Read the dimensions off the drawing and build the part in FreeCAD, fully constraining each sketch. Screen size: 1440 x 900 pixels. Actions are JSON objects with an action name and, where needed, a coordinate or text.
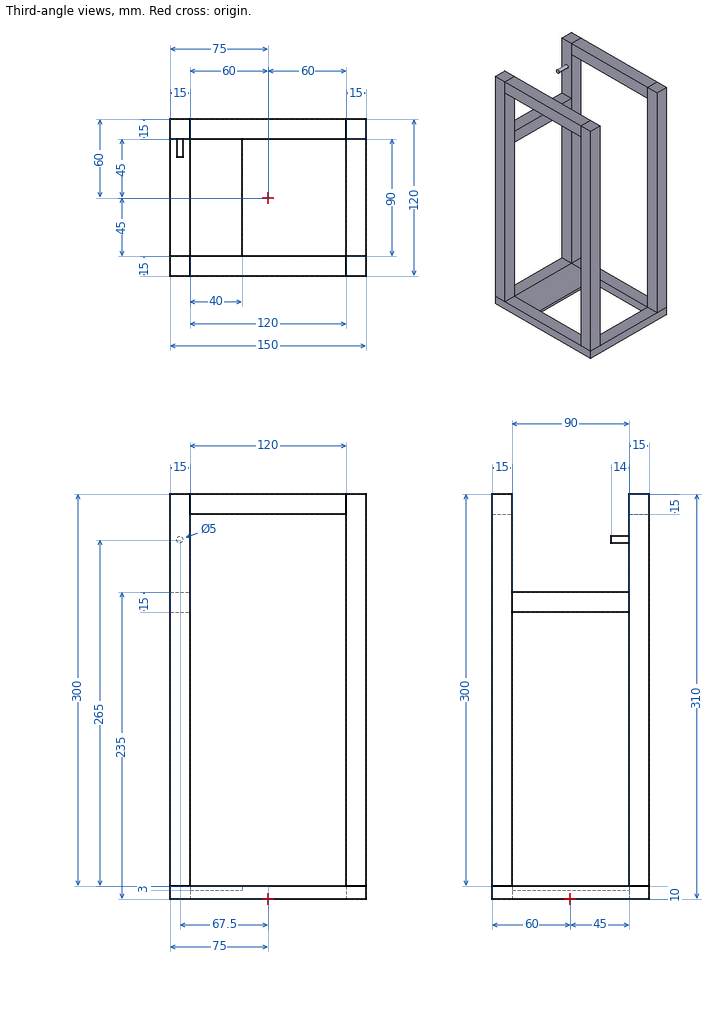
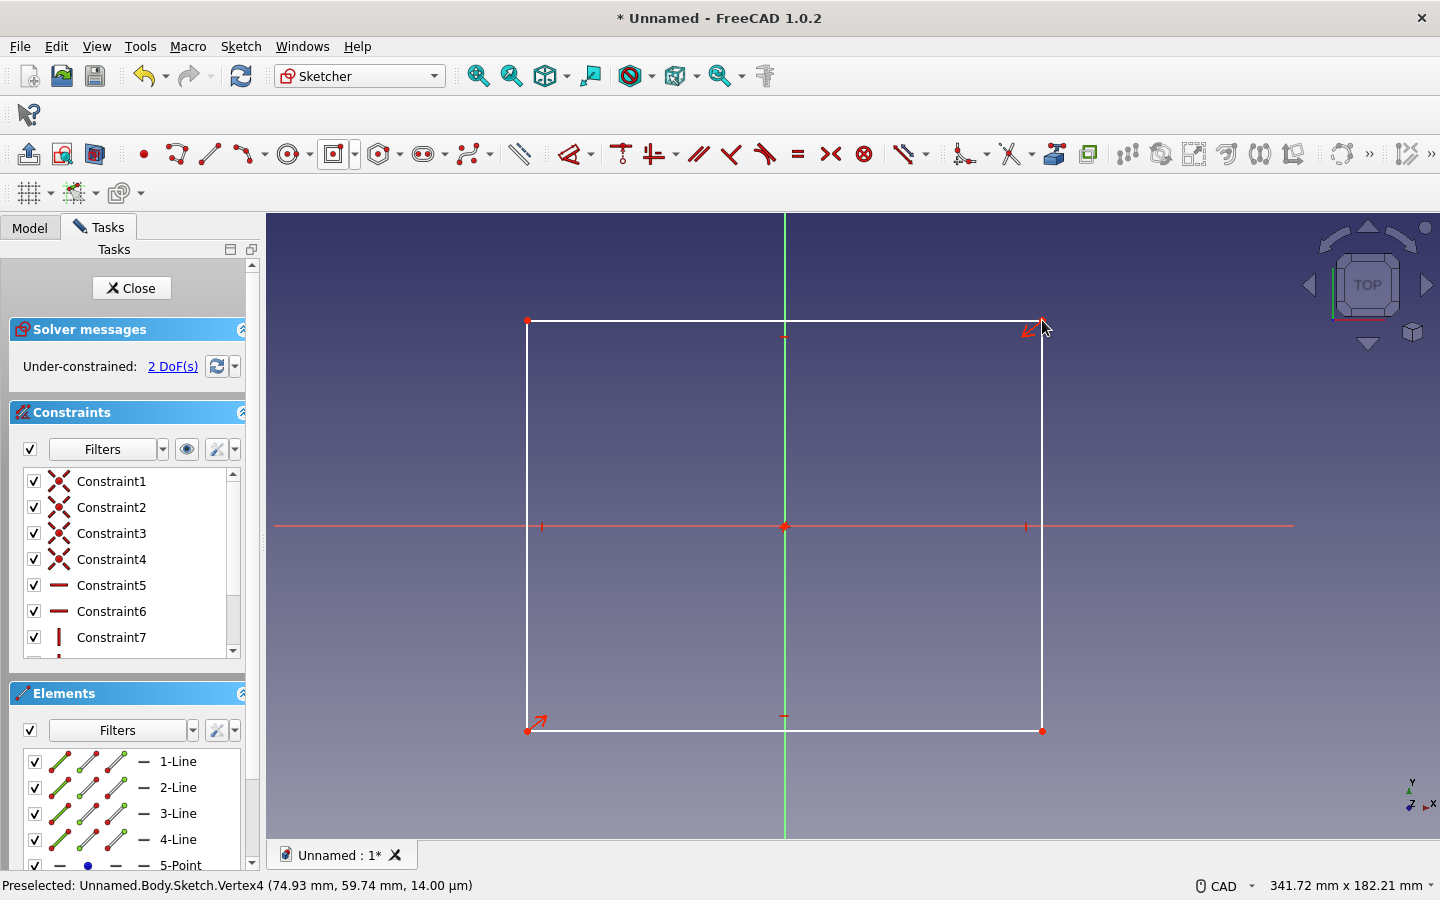
{"action": "left_click", "coordinate": [568, 154]}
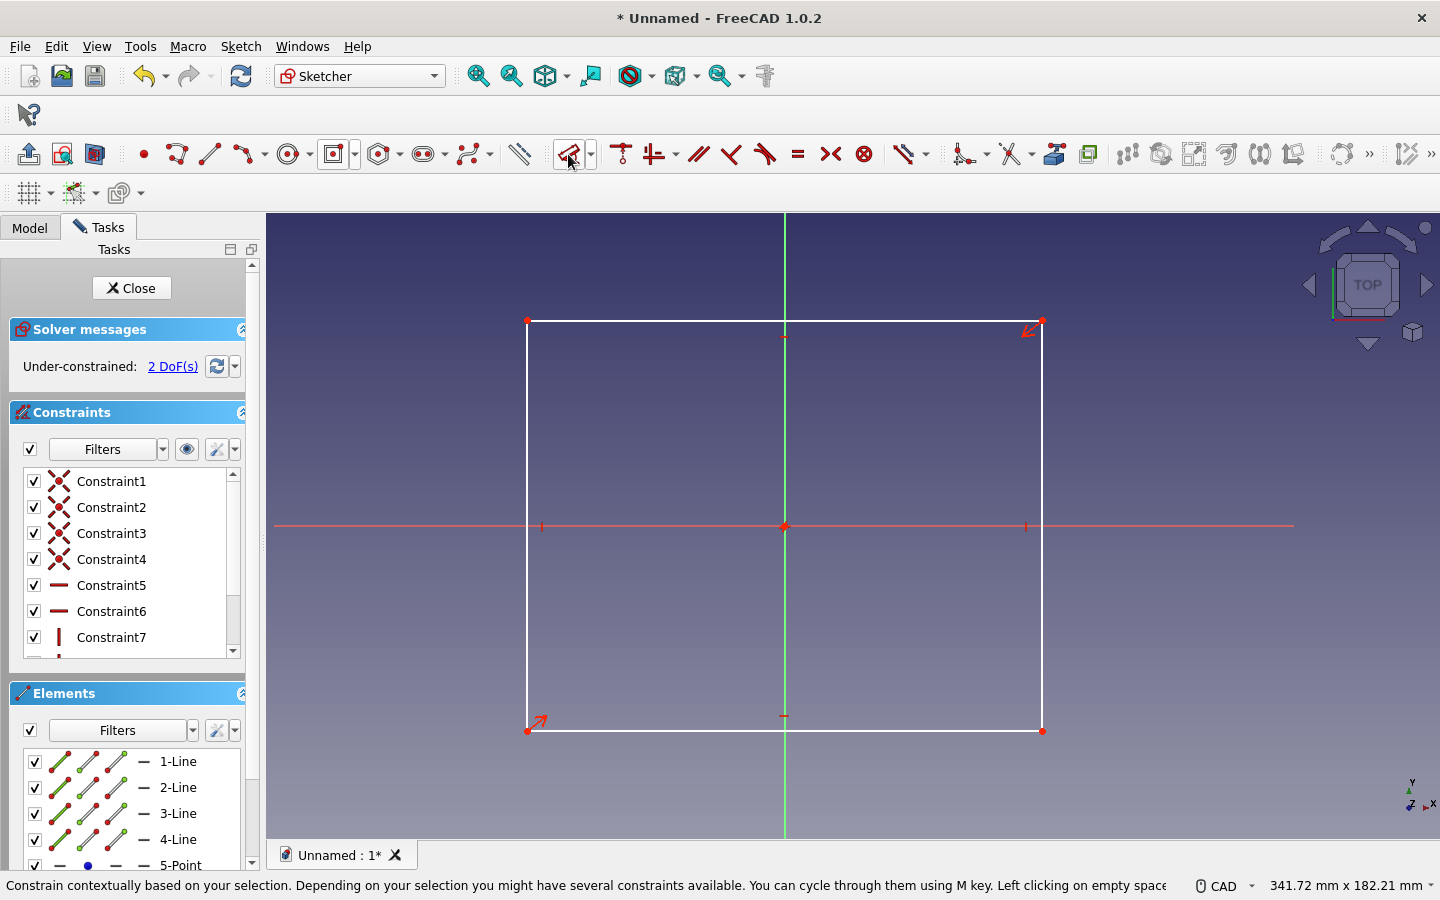
{"action": "left_click", "coordinate": [682, 731]}
{"action": "left_click", "coordinate": [666, 765]}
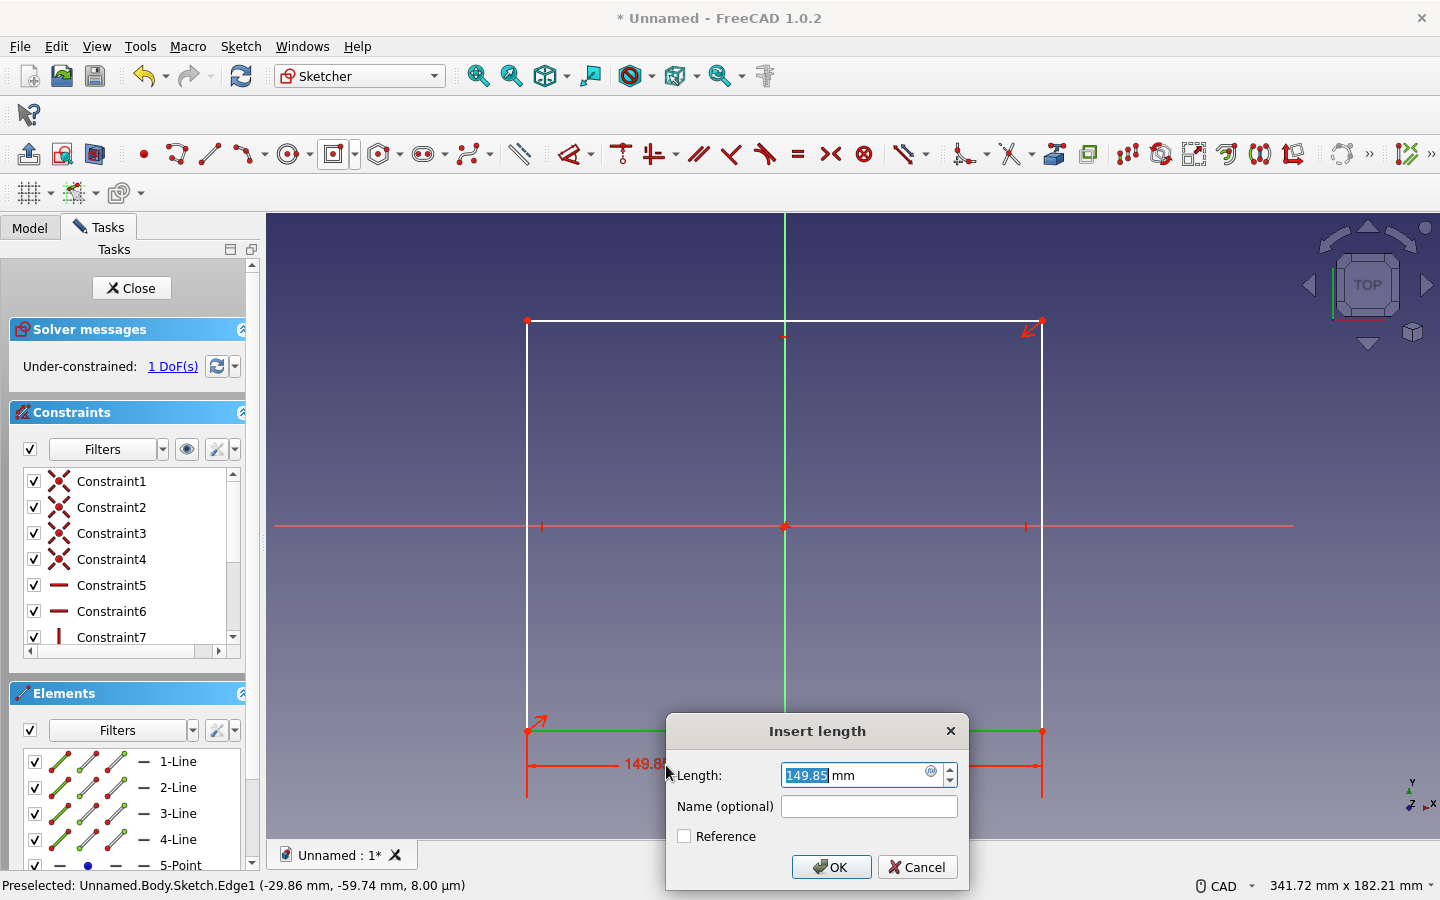
{"action": "type", "text": "150"}
{"action": "key", "text": "Return"}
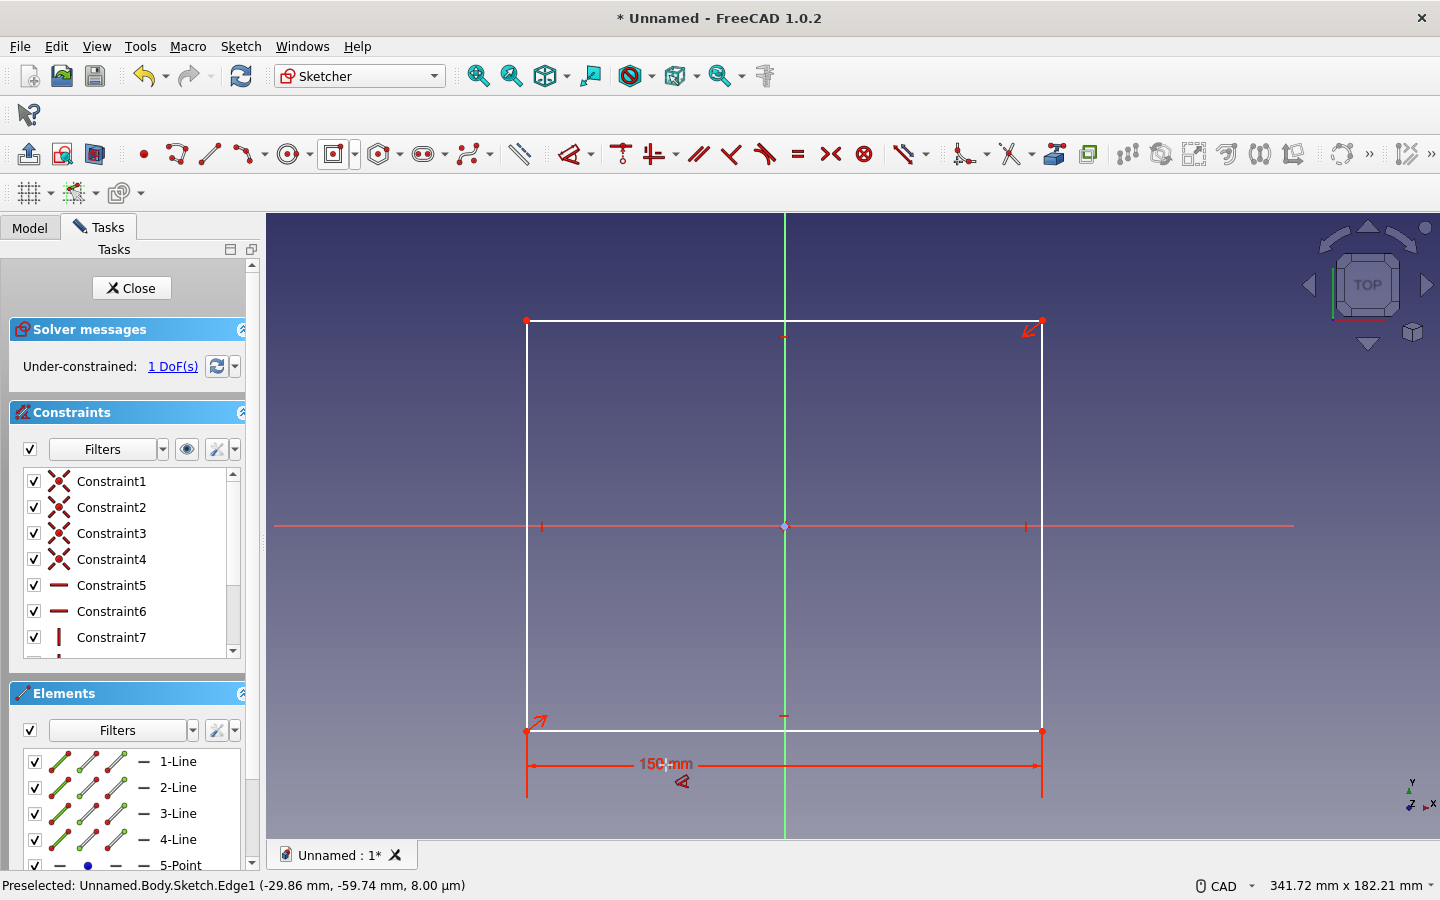
{"action": "left_click", "coordinate": [1042, 608]}
{"action": "left_click", "coordinate": [1076, 432]}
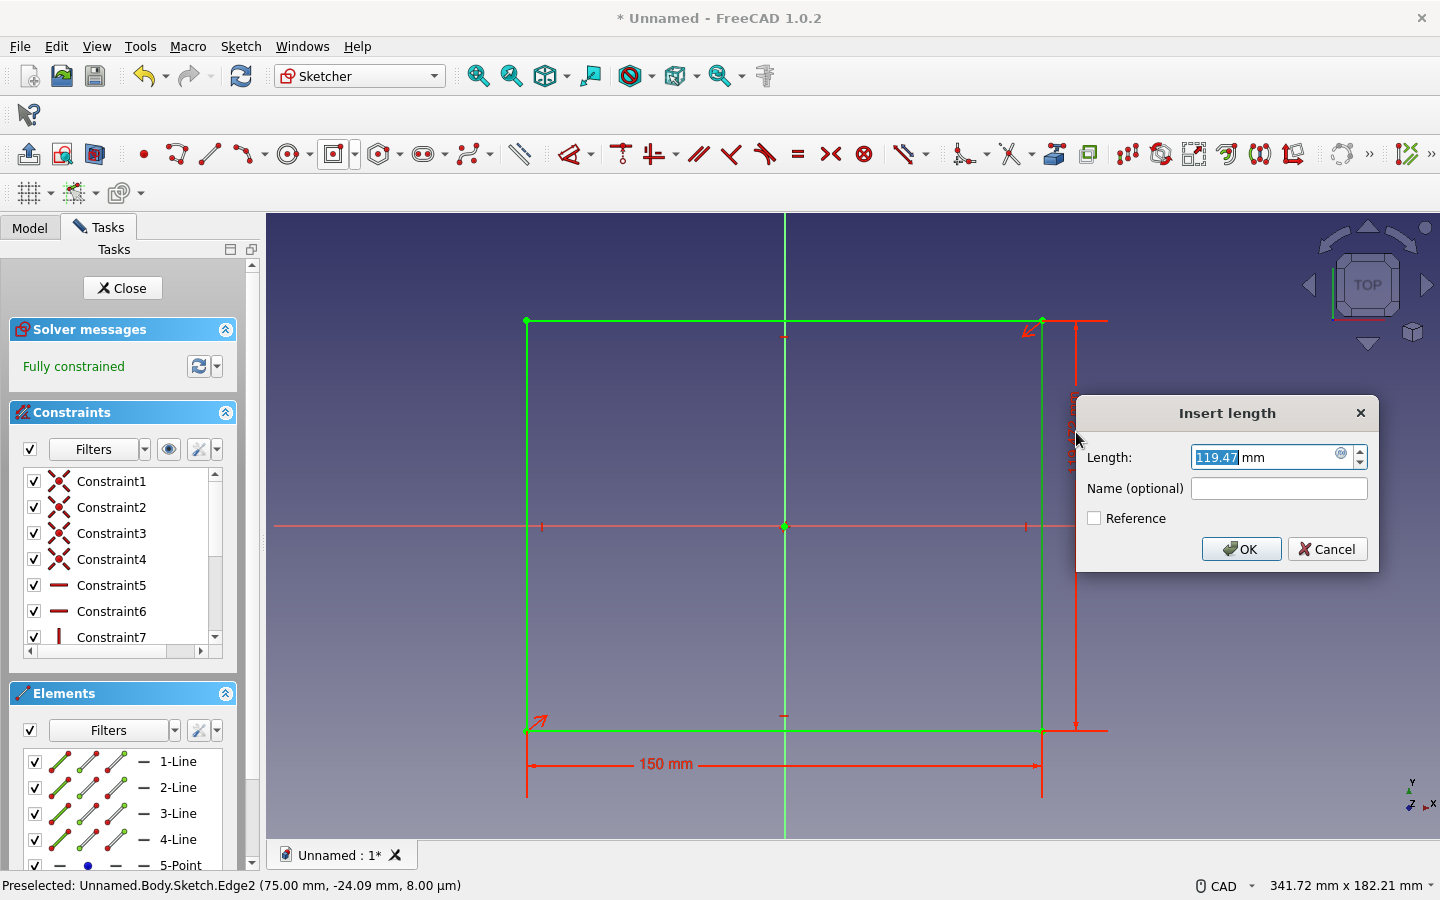
{"action": "type", "text": "120"}
{"action": "key", "text": "Return"}
{"action": "key", "text": "Escape"}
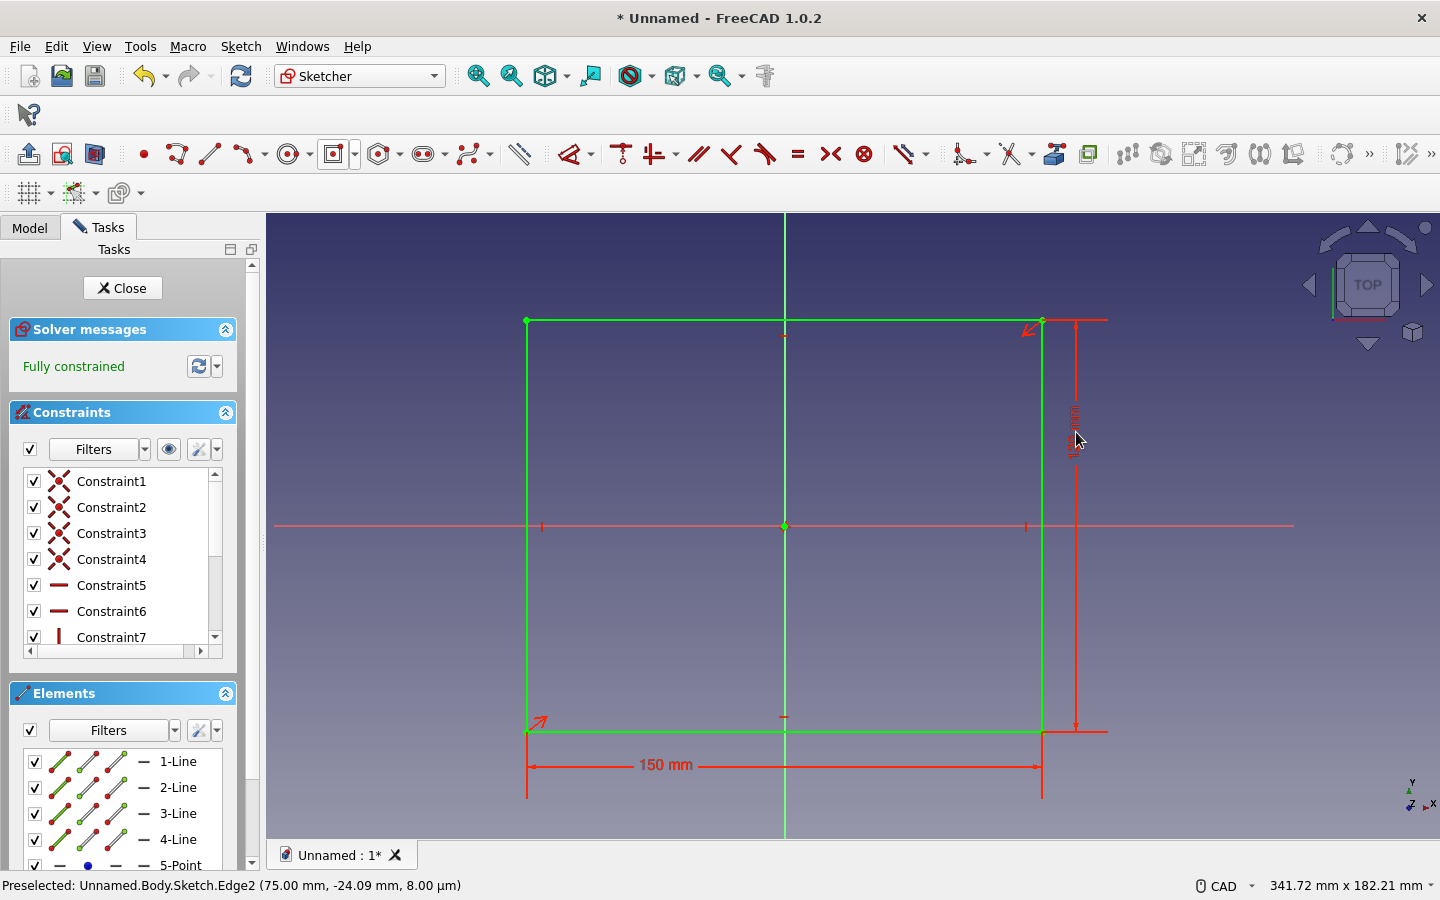
{"action": "left_click", "coordinate": [123, 288]}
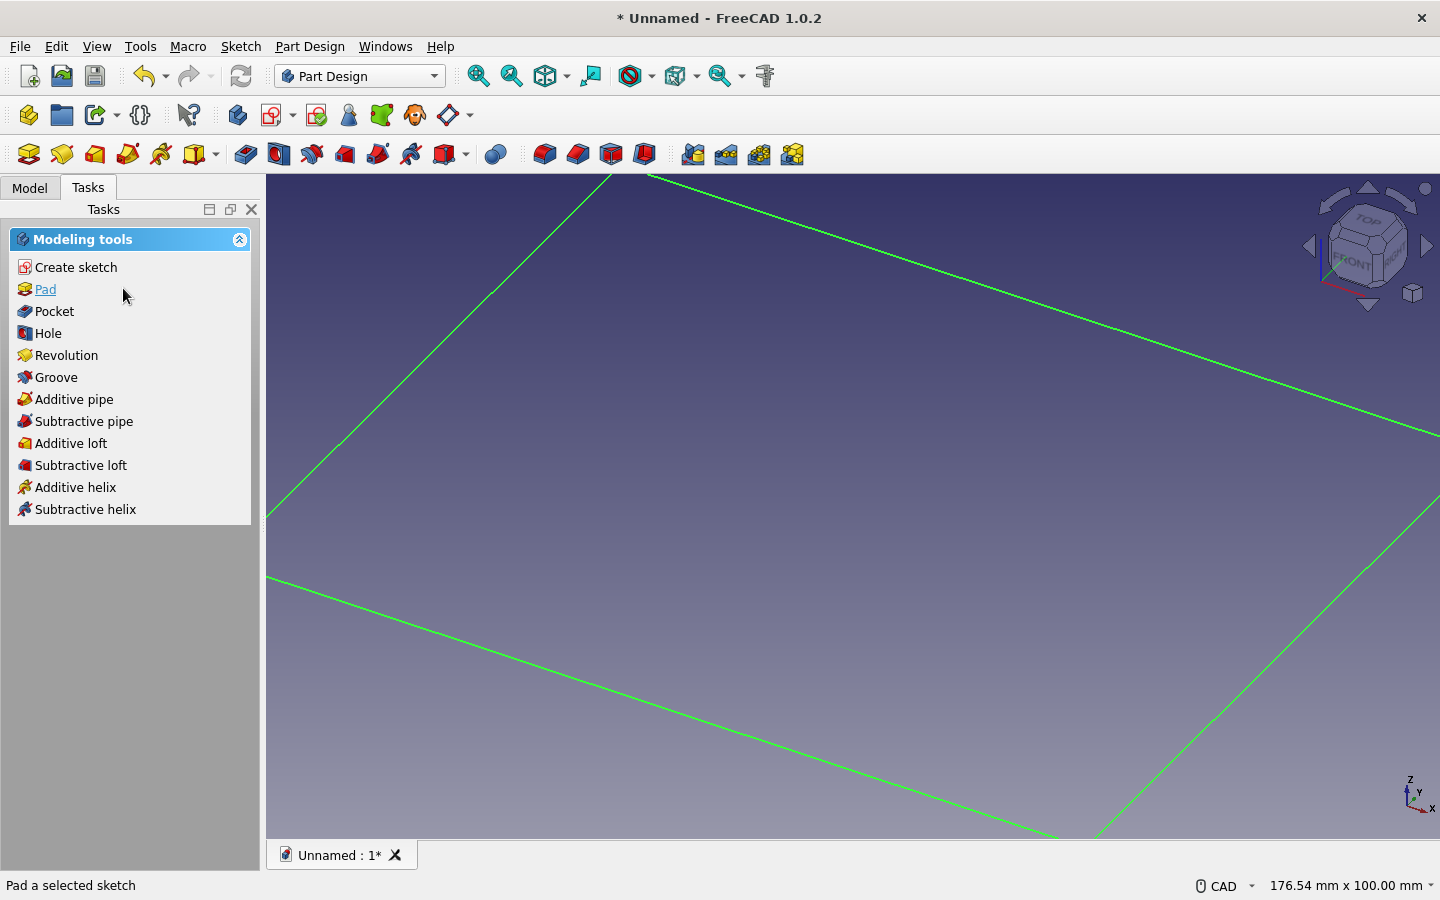
{"action": "left_click", "coordinate": [29, 154]}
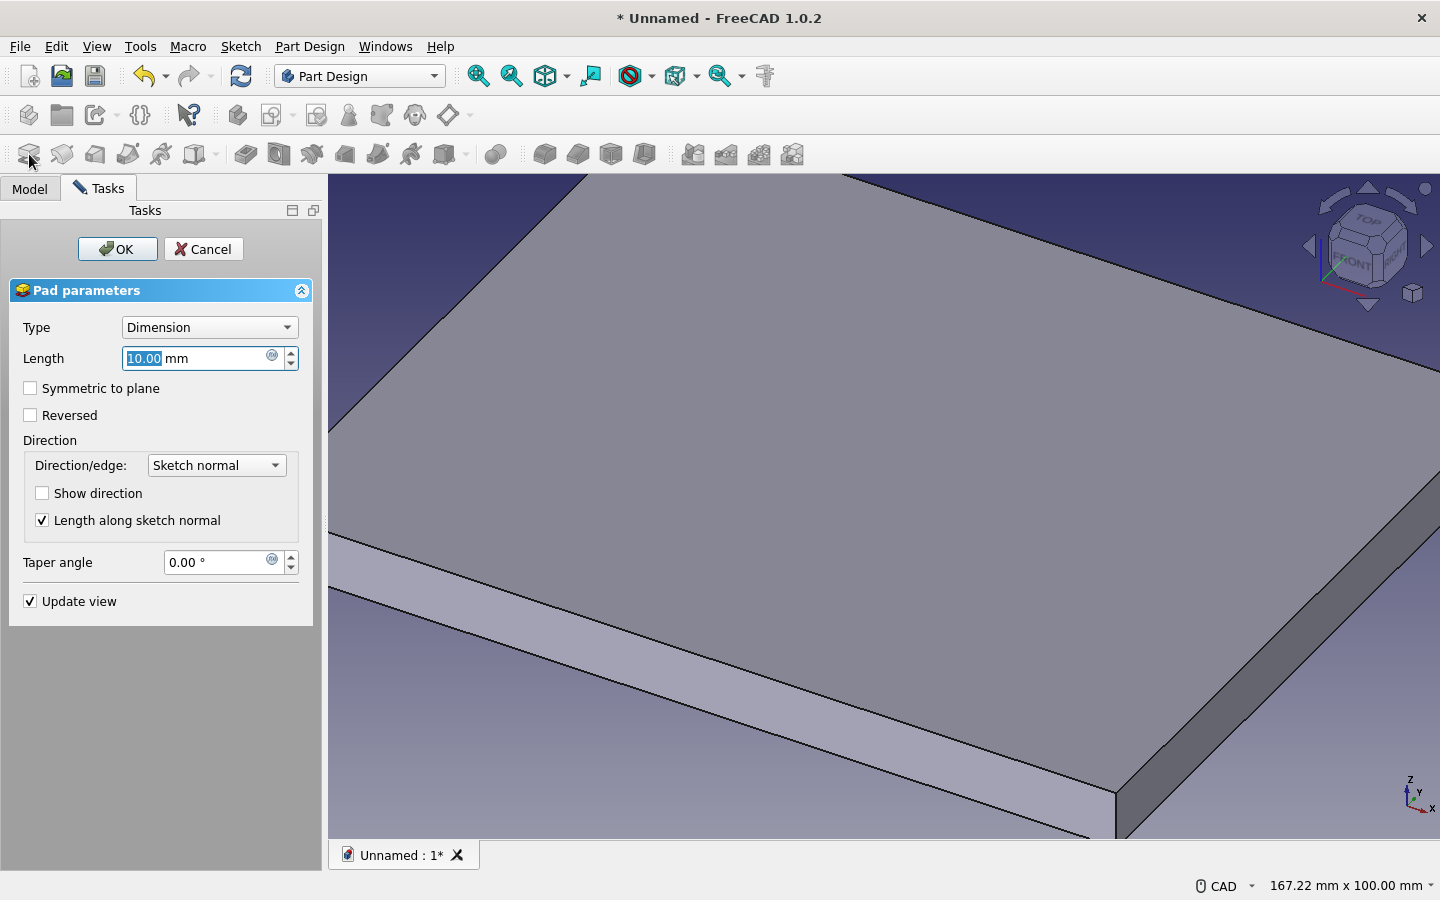
{"action": "type", "text": "10"}
{"action": "key", "text": "Tab"}